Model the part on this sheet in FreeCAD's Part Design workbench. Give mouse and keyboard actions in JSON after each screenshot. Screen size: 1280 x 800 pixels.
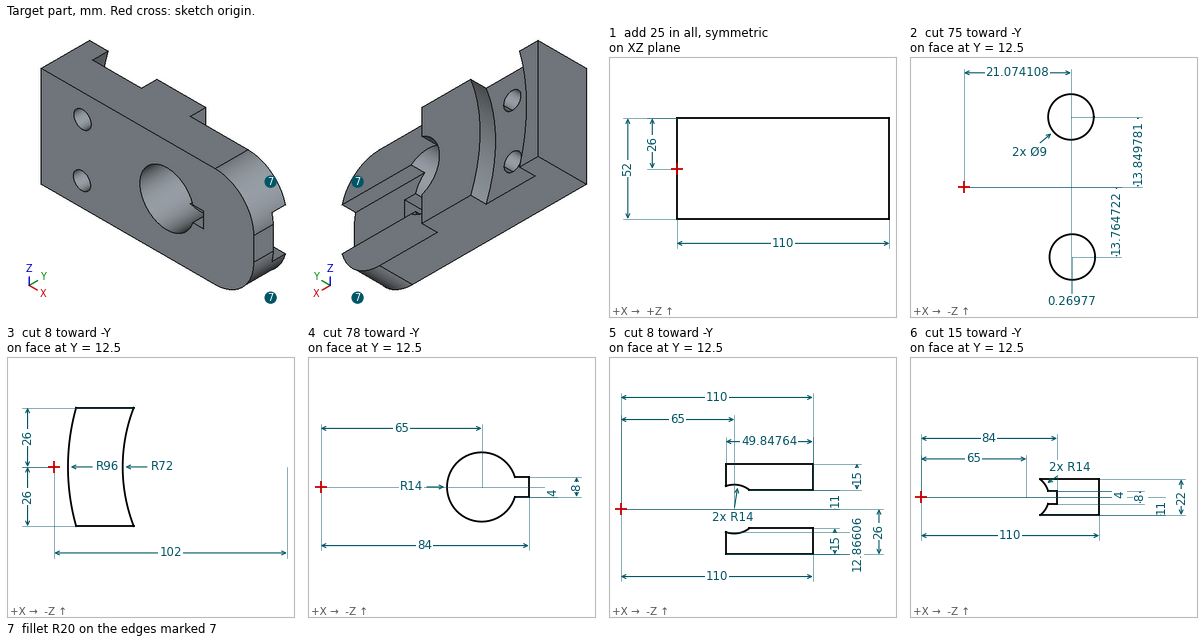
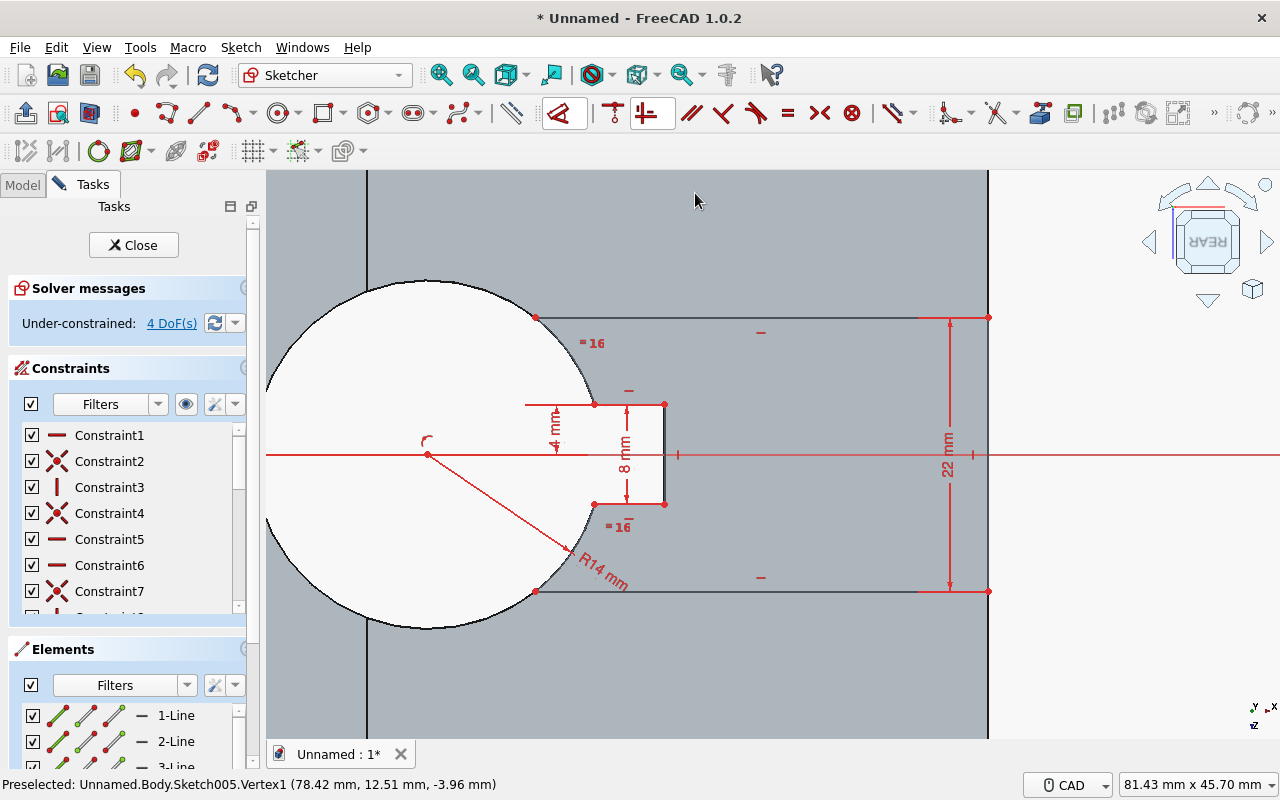
{"action": "left_click", "coordinate": [665, 405]}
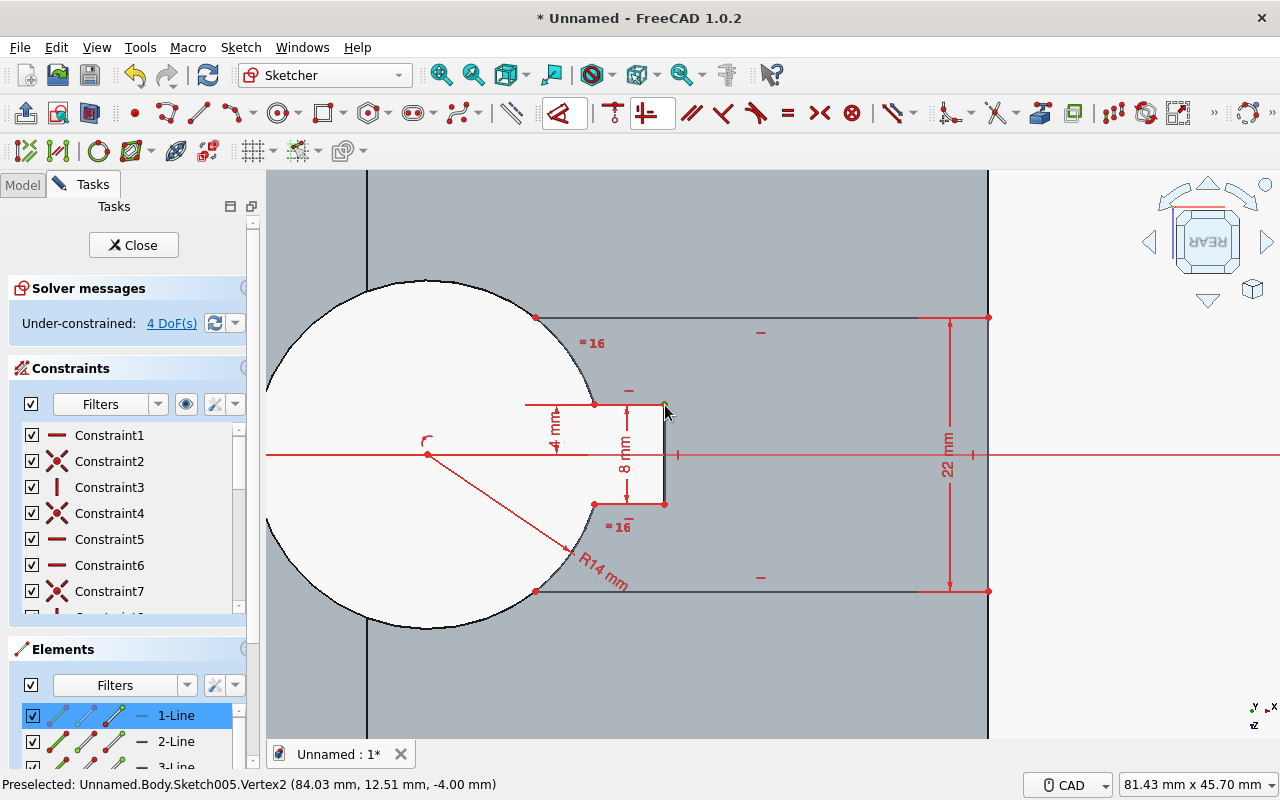
{"action": "key", "text": "l"}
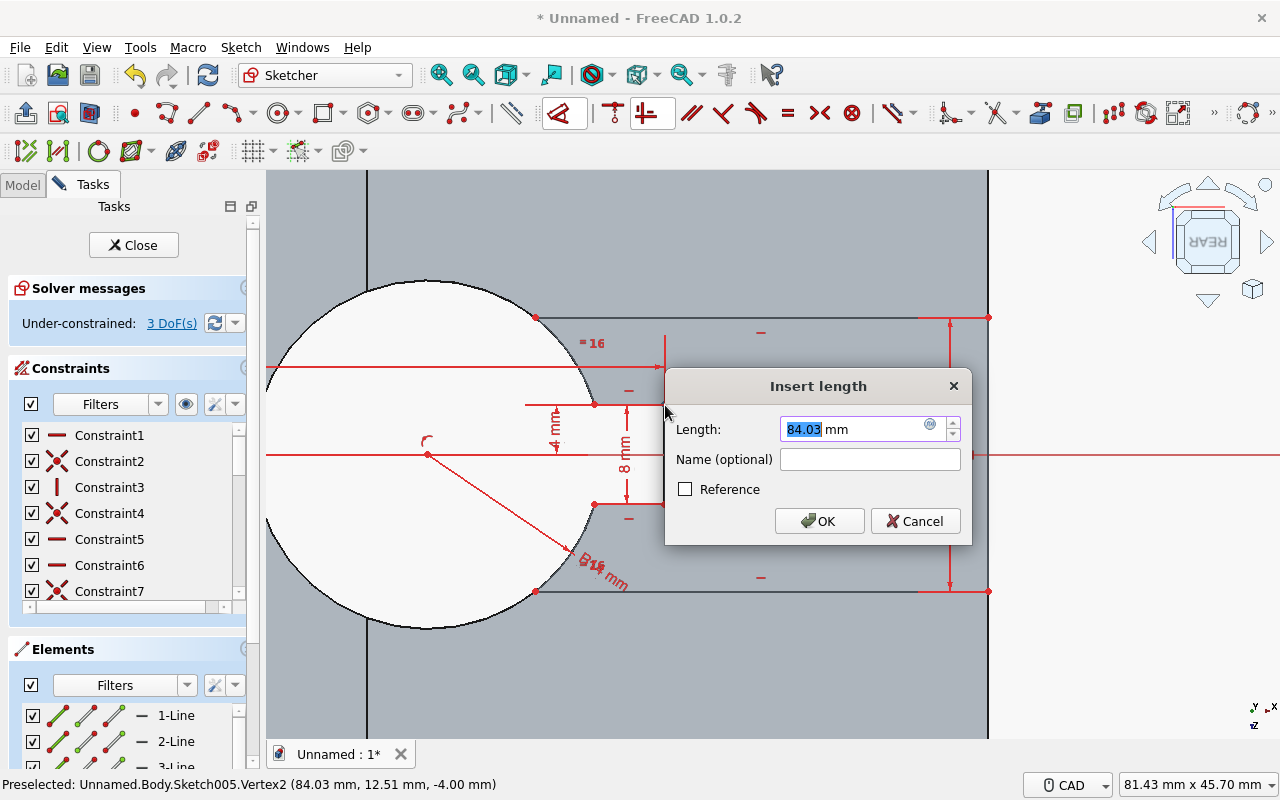
{"action": "type", "text": "84"}
{"action": "key", "text": "Return"}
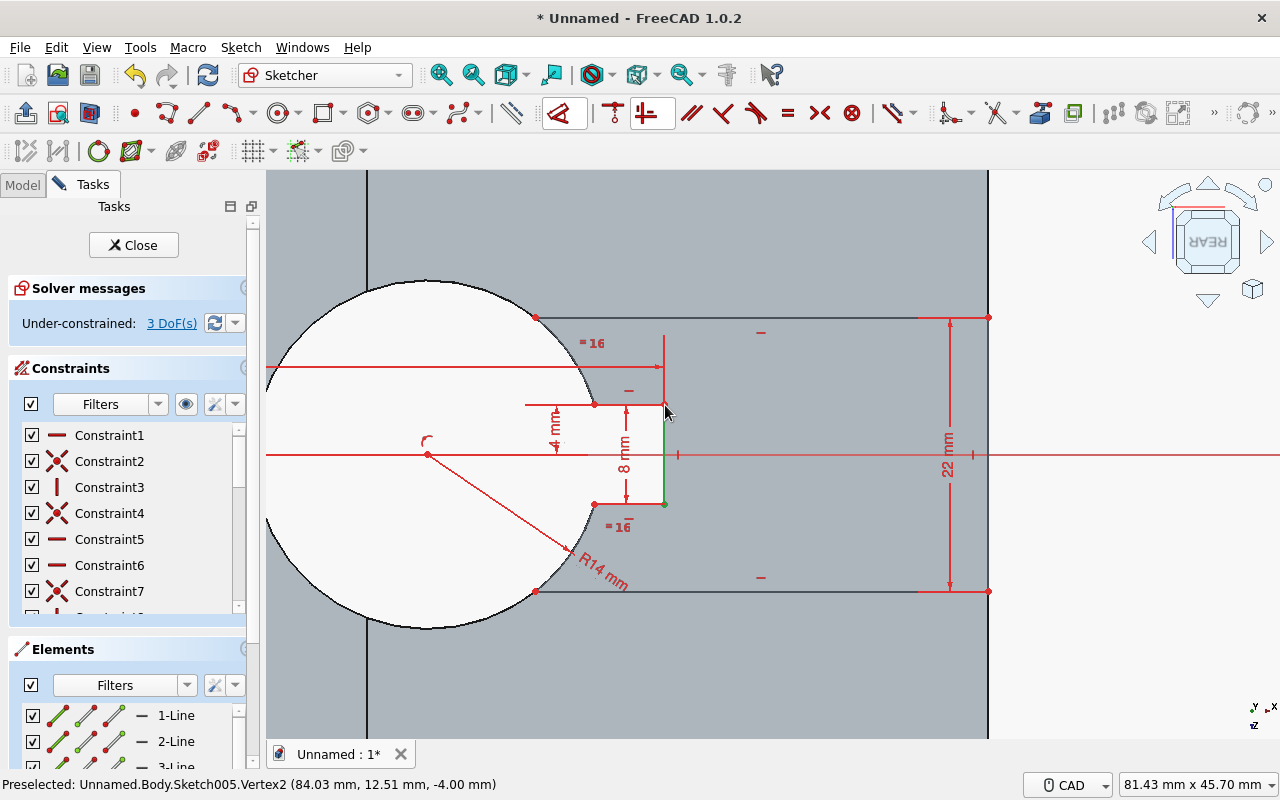
{"action": "left_click", "coordinate": [535, 592]}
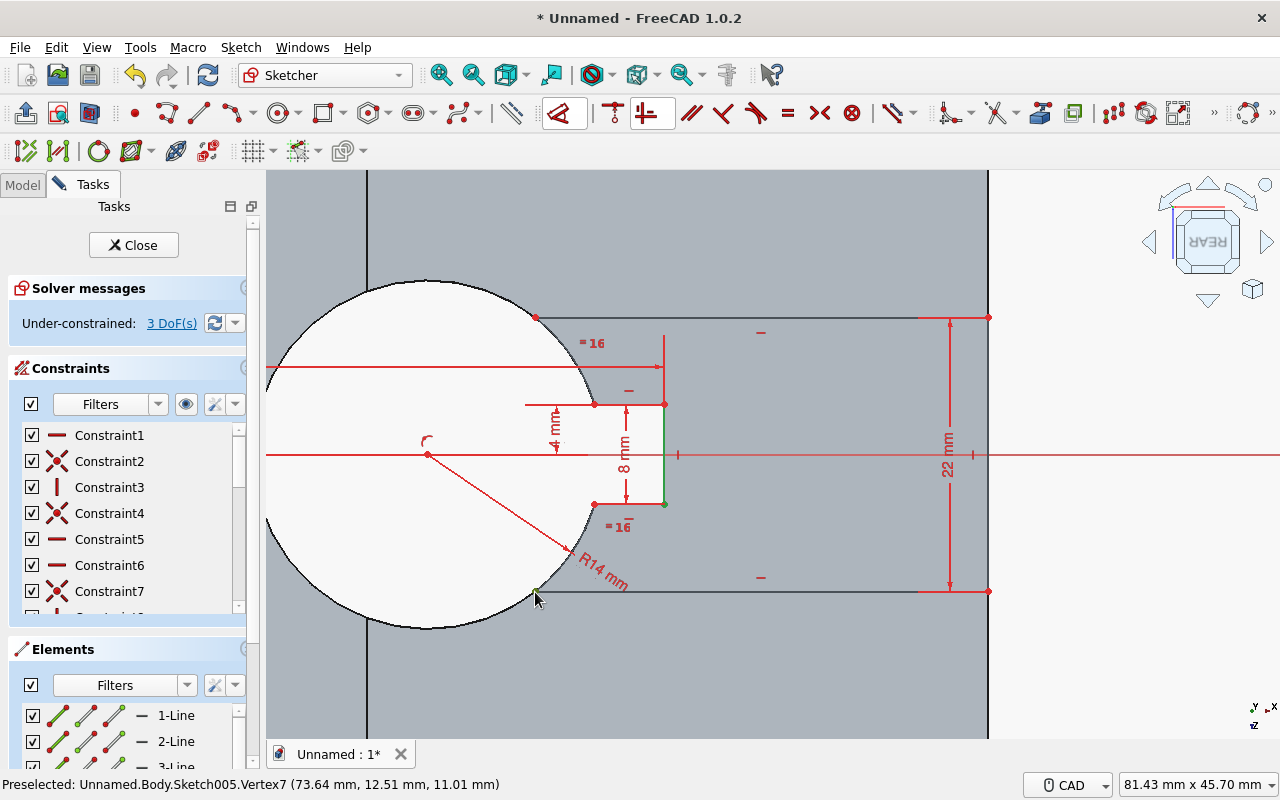
{"action": "left_click", "coordinate": [582, 114]}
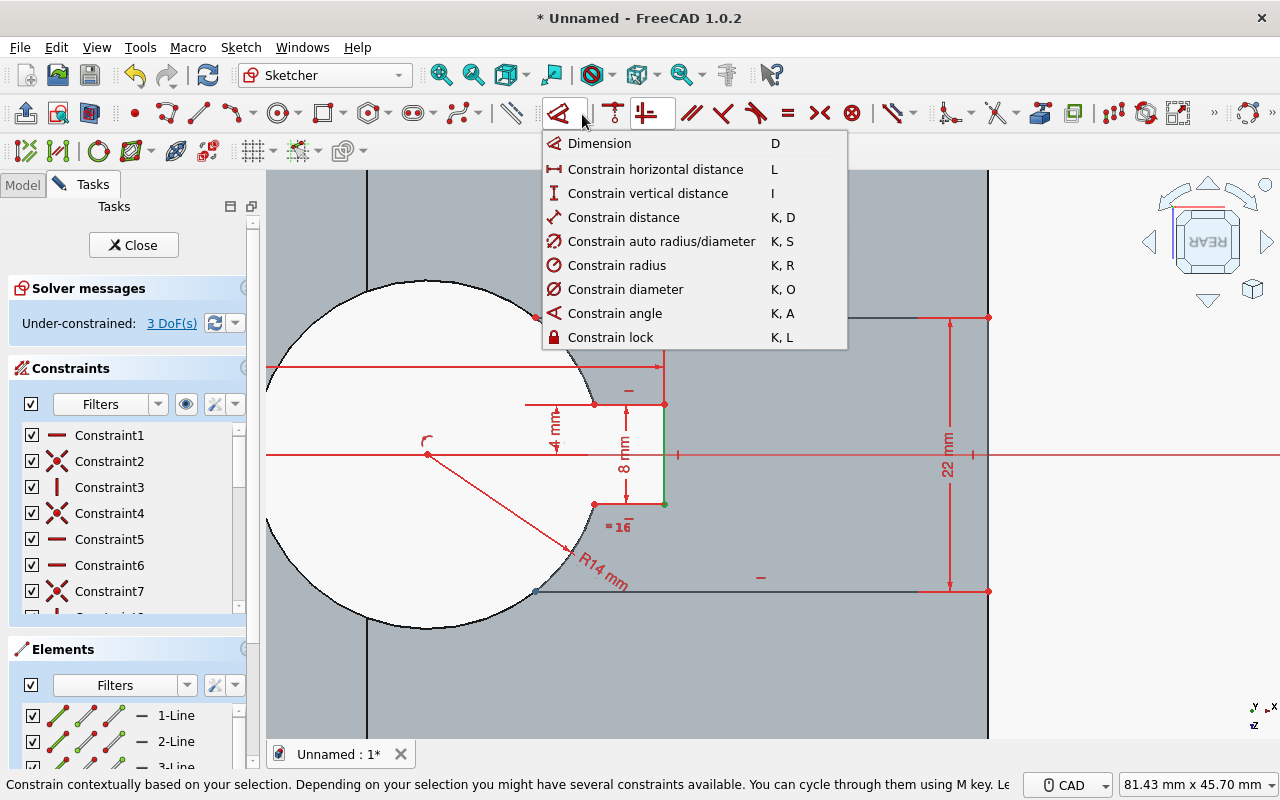
{"action": "left_click", "coordinate": [695, 193]}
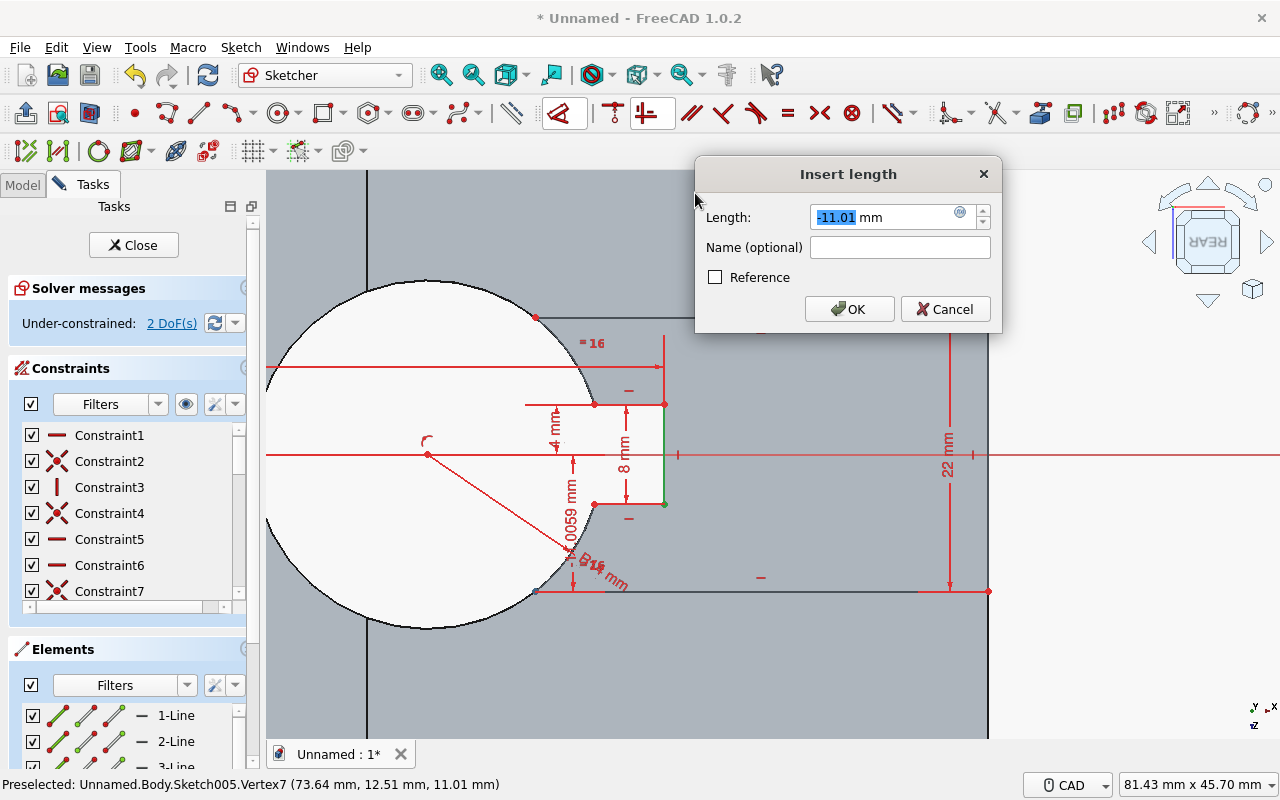
{"action": "type", "text": "-11"}
{"action": "key", "text": "Return"}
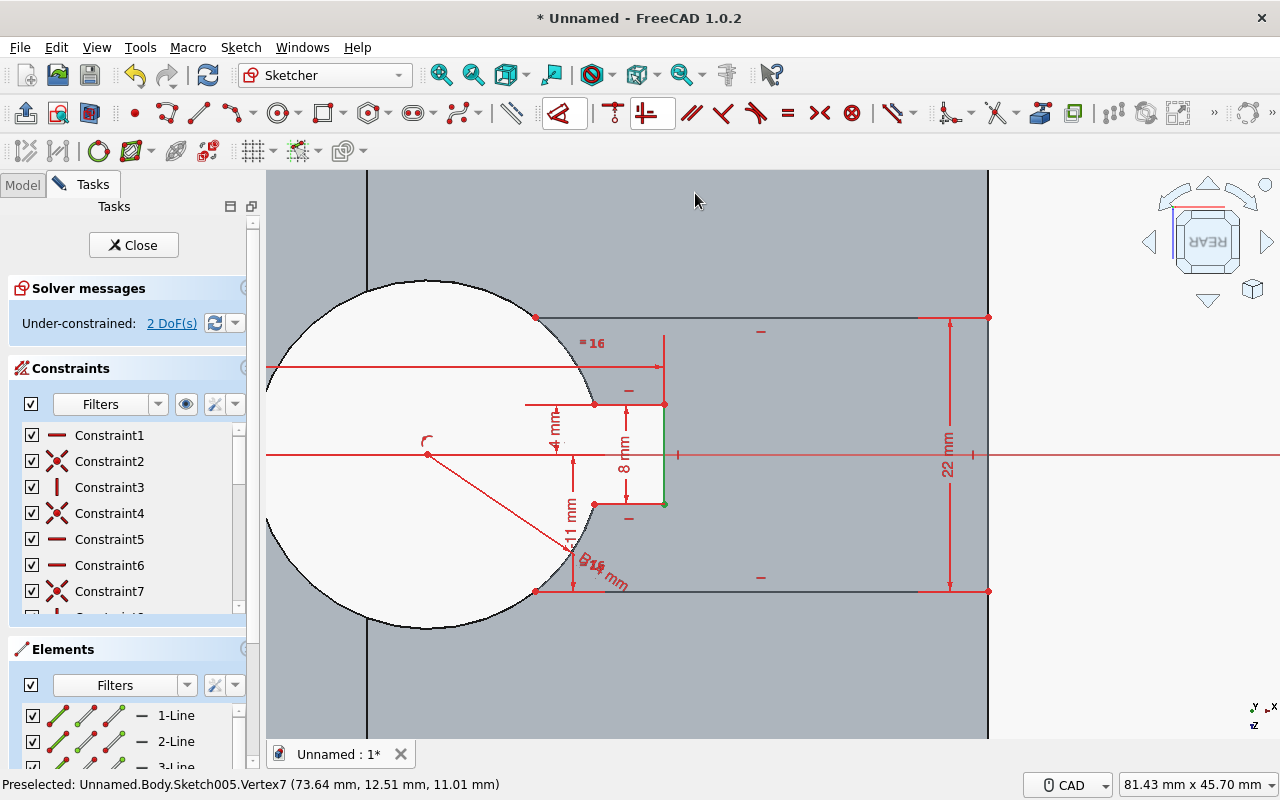
{"action": "left_click", "coordinate": [427, 455]}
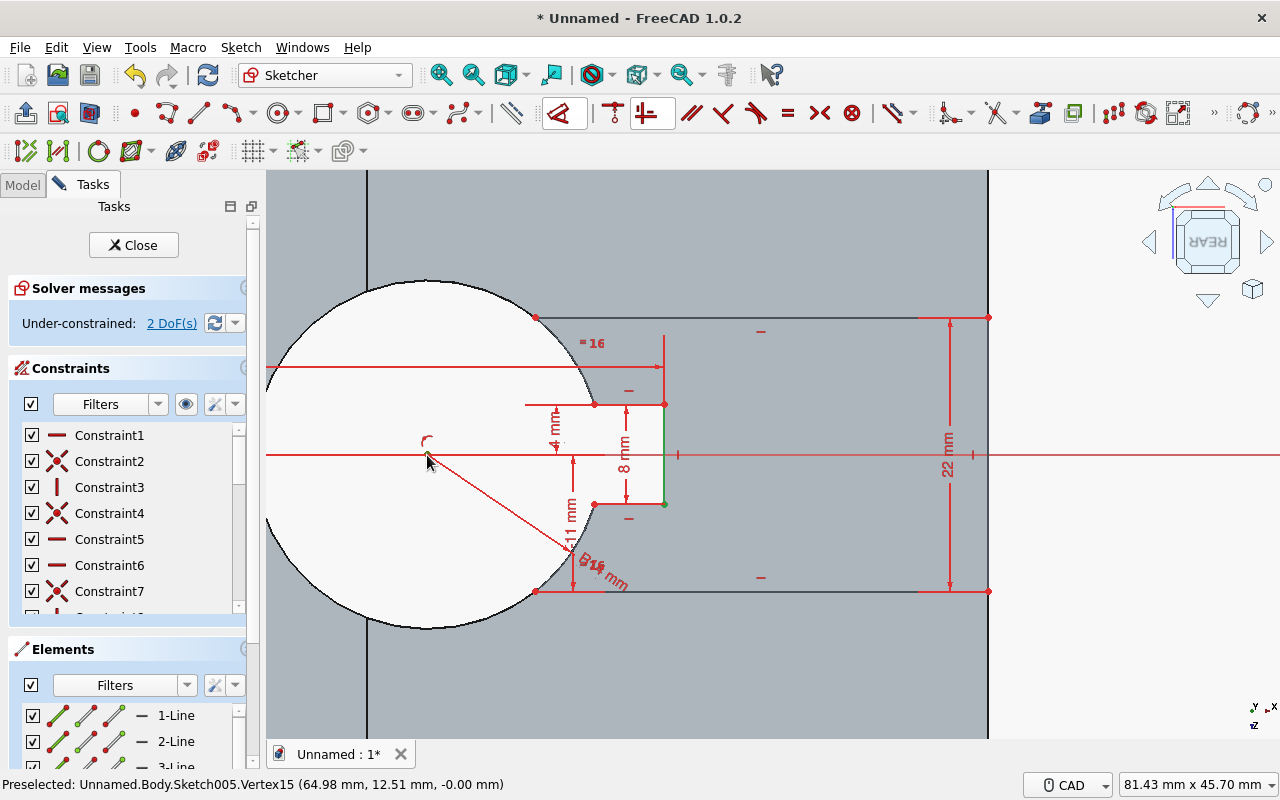
{"action": "left_click", "coordinate": [582, 114]}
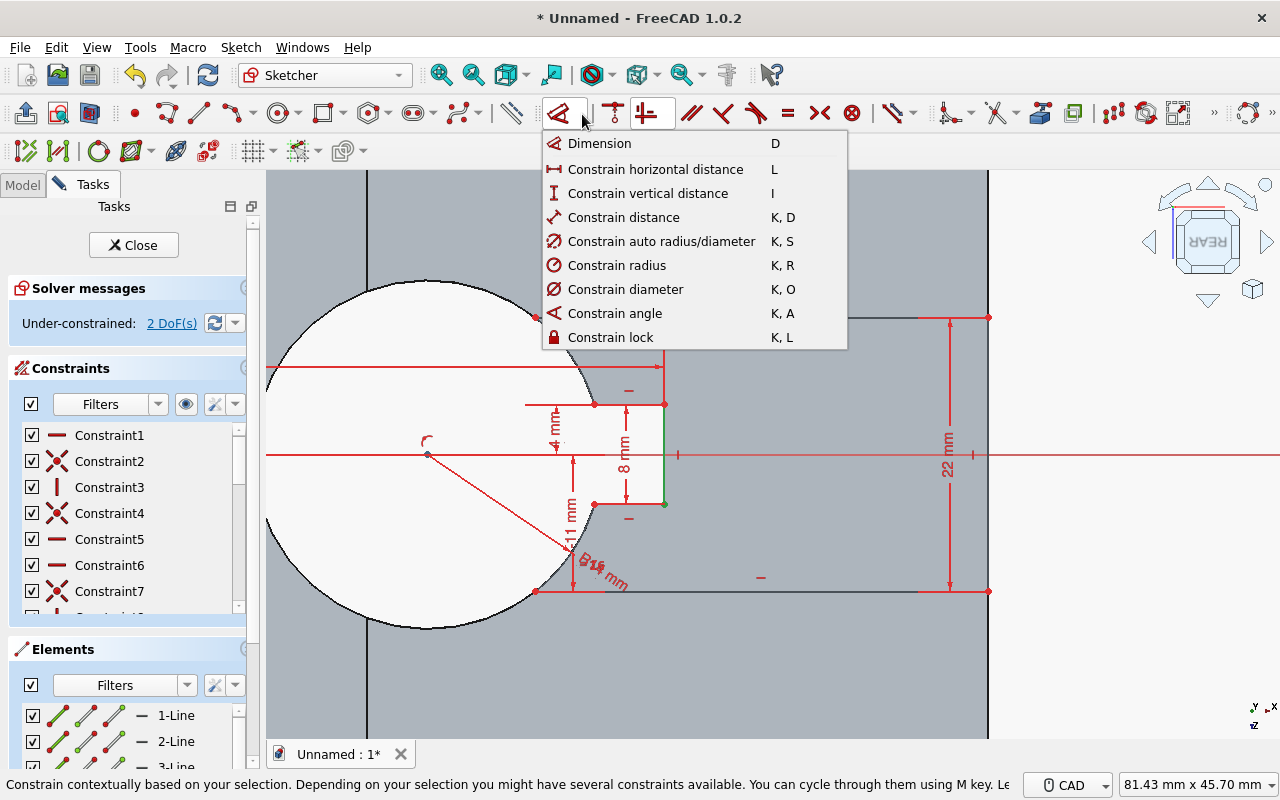
{"action": "left_click", "coordinate": [695, 169]}